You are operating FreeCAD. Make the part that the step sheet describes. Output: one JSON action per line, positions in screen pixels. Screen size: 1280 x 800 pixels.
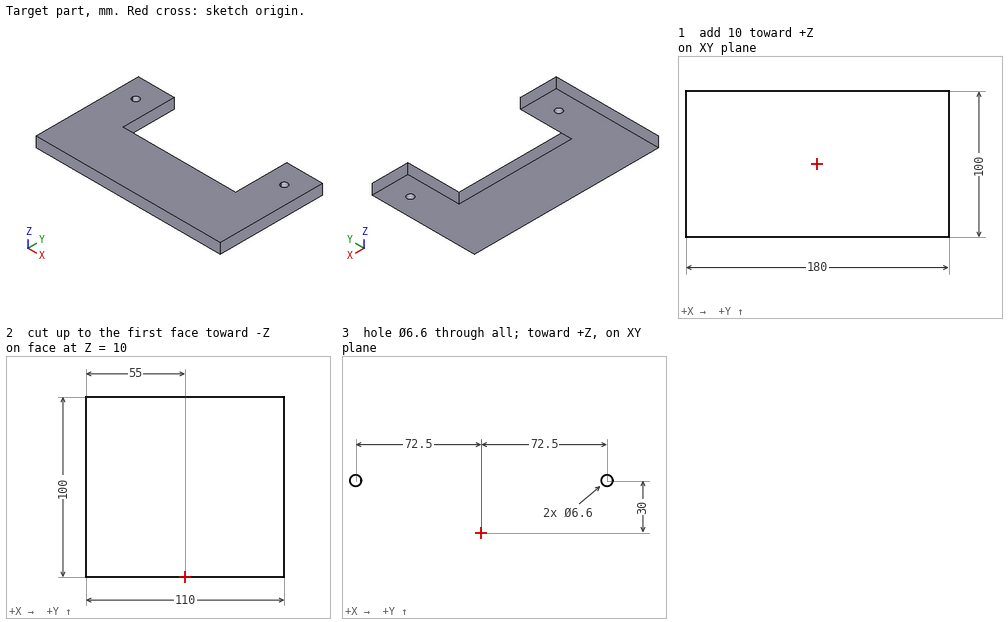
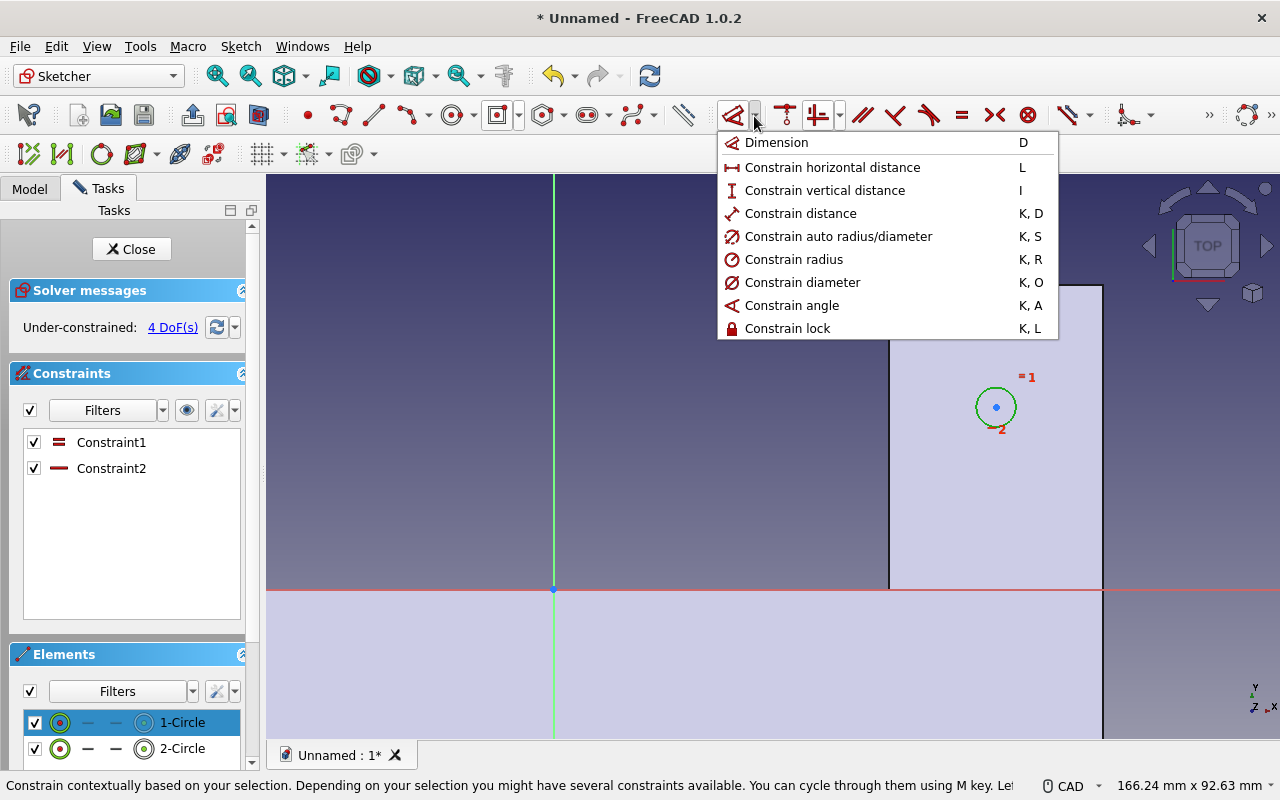
{"action": "left_click", "coordinate": [888, 282]}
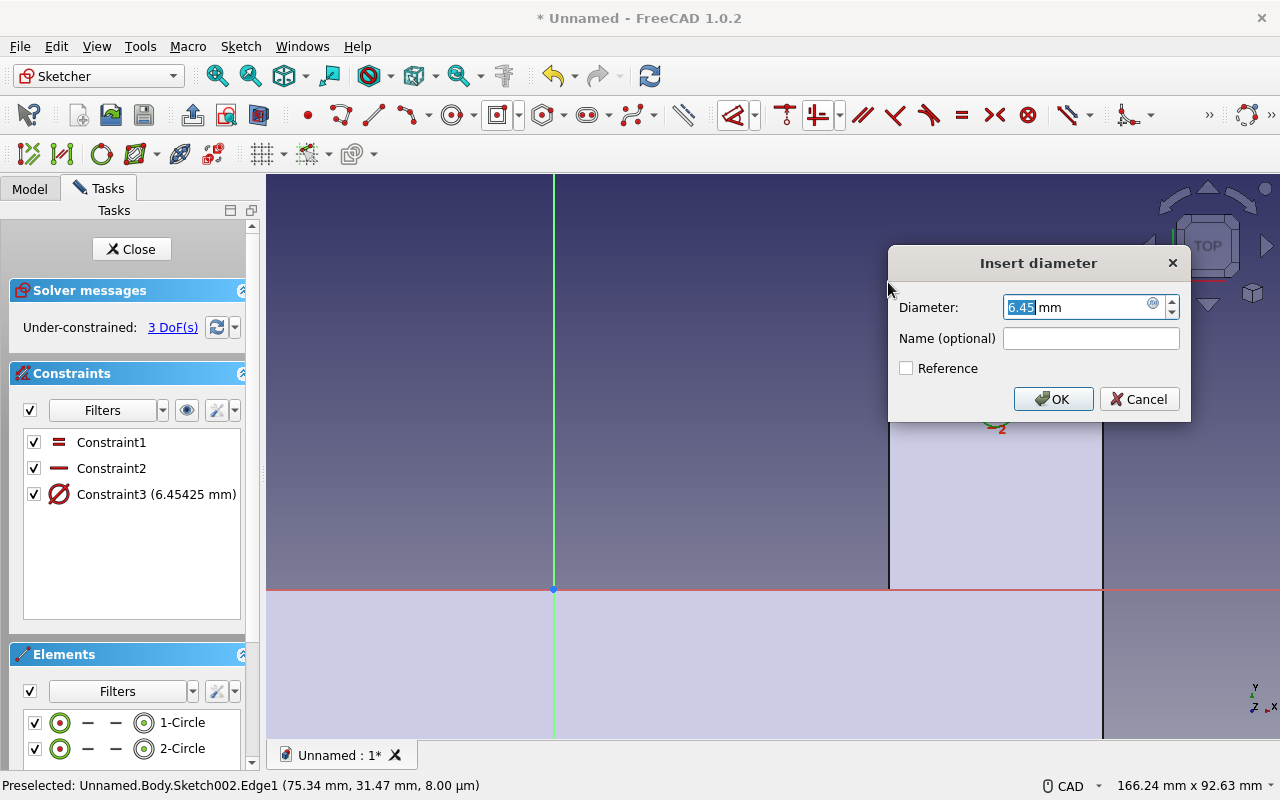
{"action": "type", "text": "6.6"}
{"action": "key", "text": "Return"}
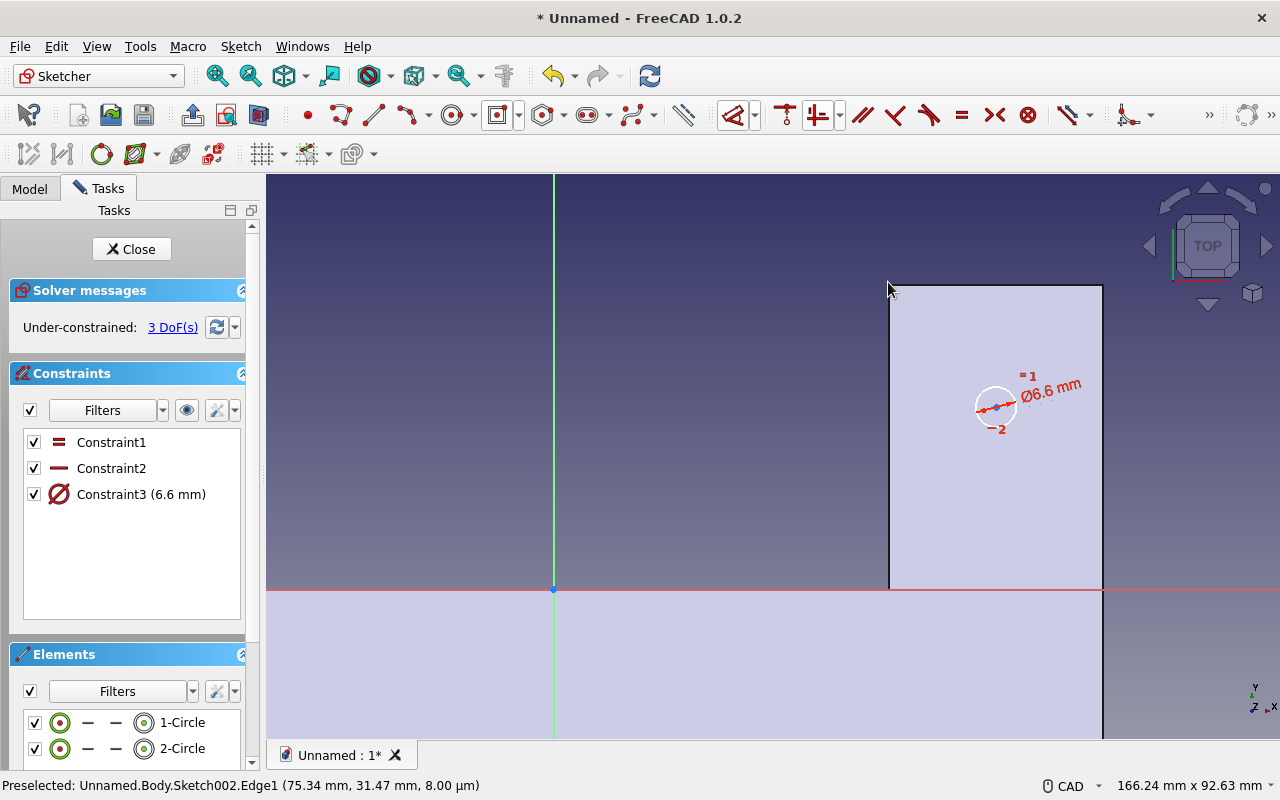
{"action": "left_click", "coordinate": [996, 407]}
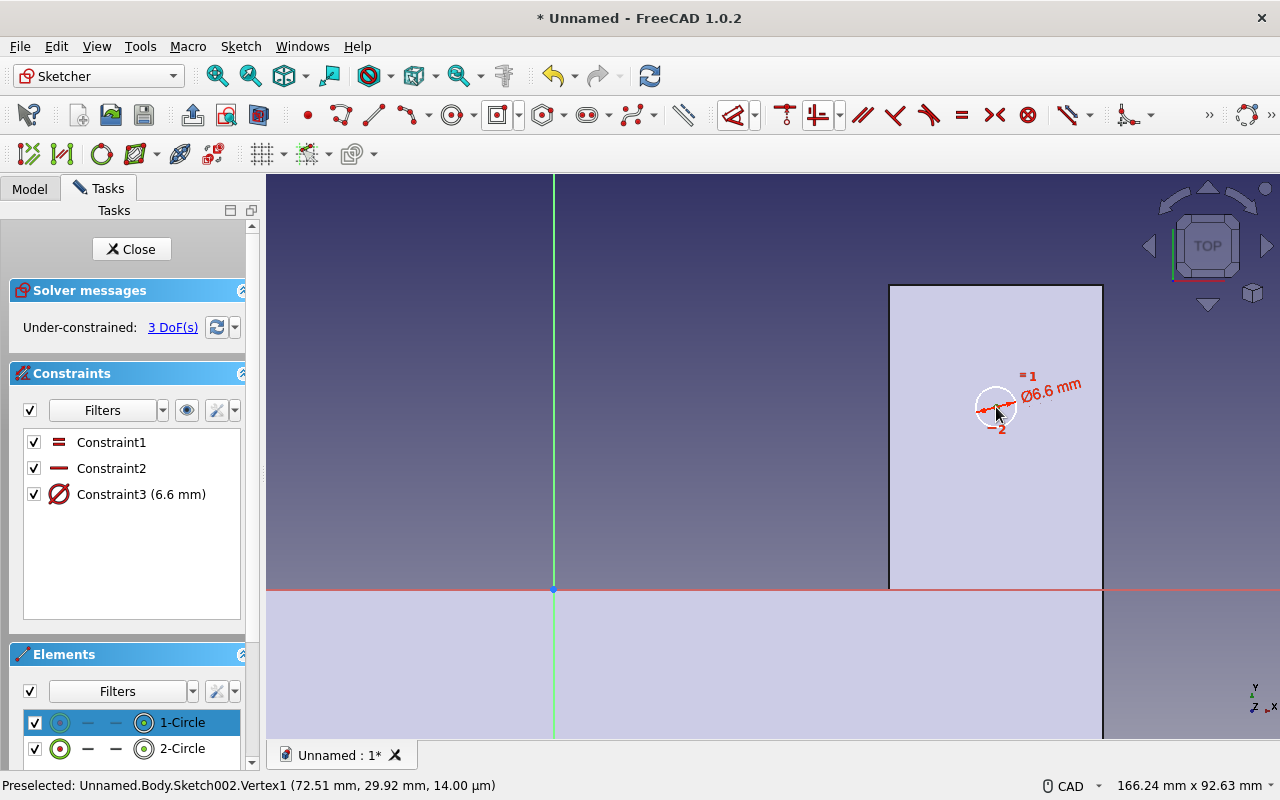
{"action": "key", "text": "i"}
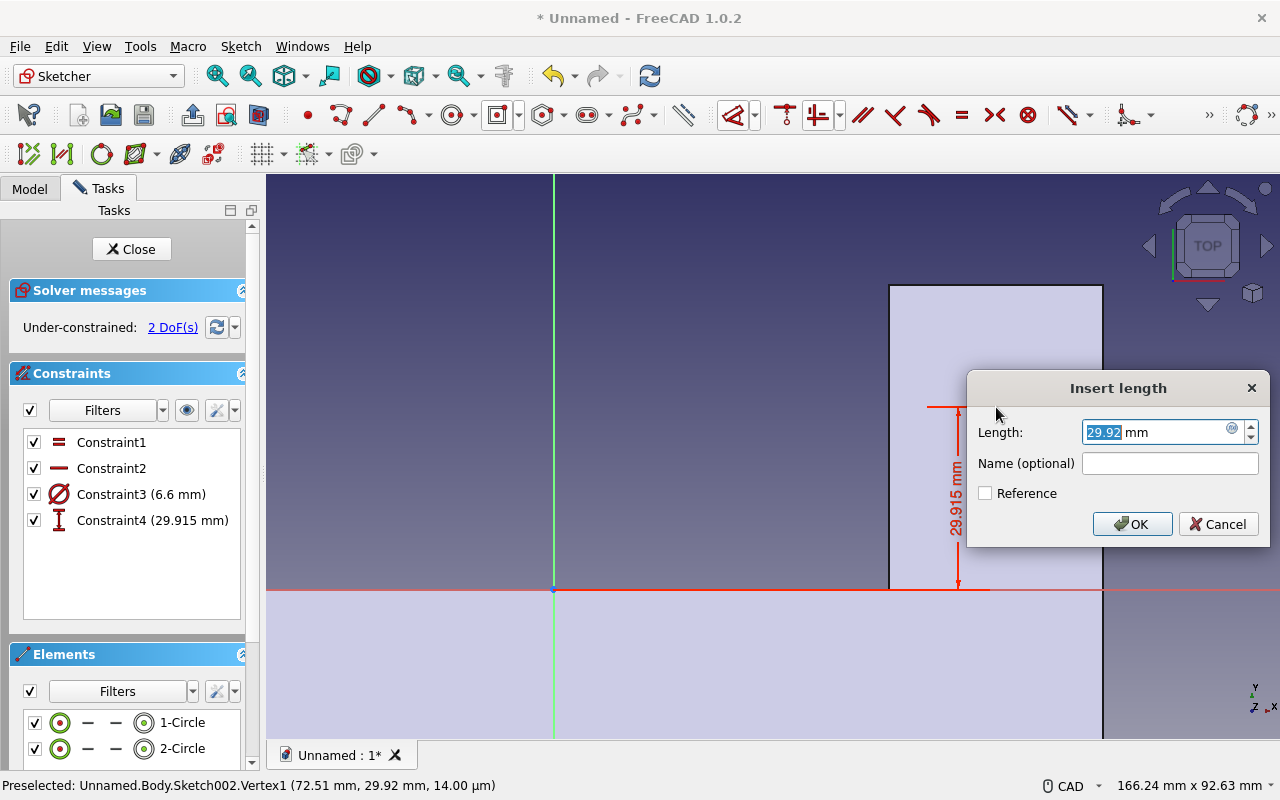
{"action": "type", "text": "30"}
{"action": "key", "text": "Return"}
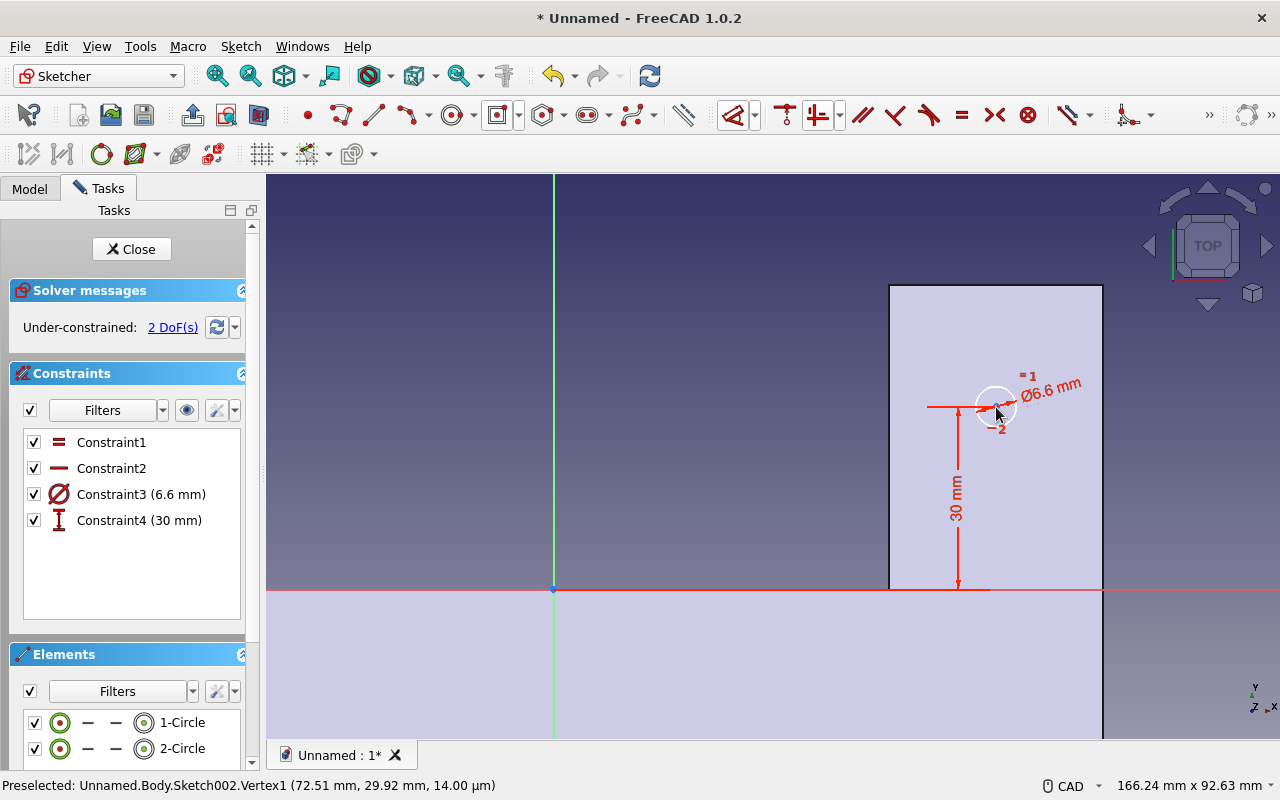
{"action": "left_click", "coordinate": [996, 407]}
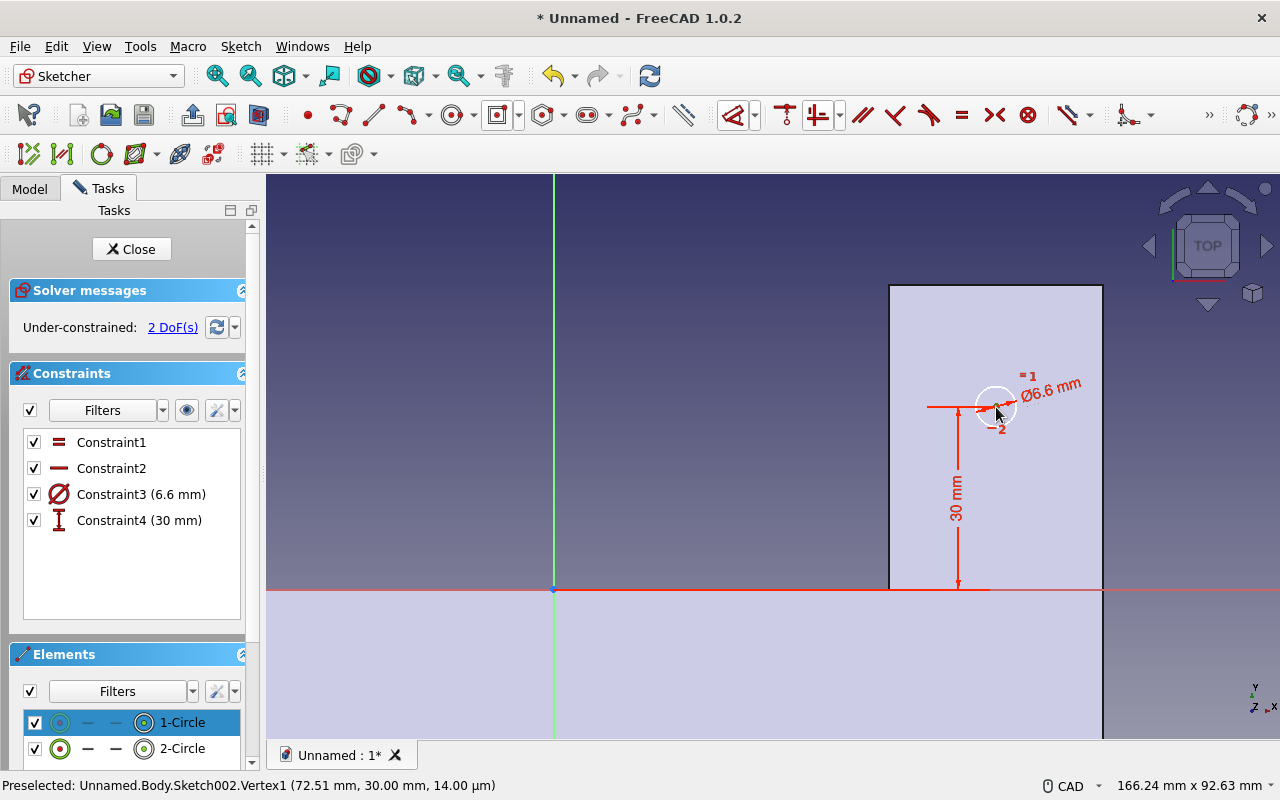
{"action": "left_click", "coordinate": [754, 116]}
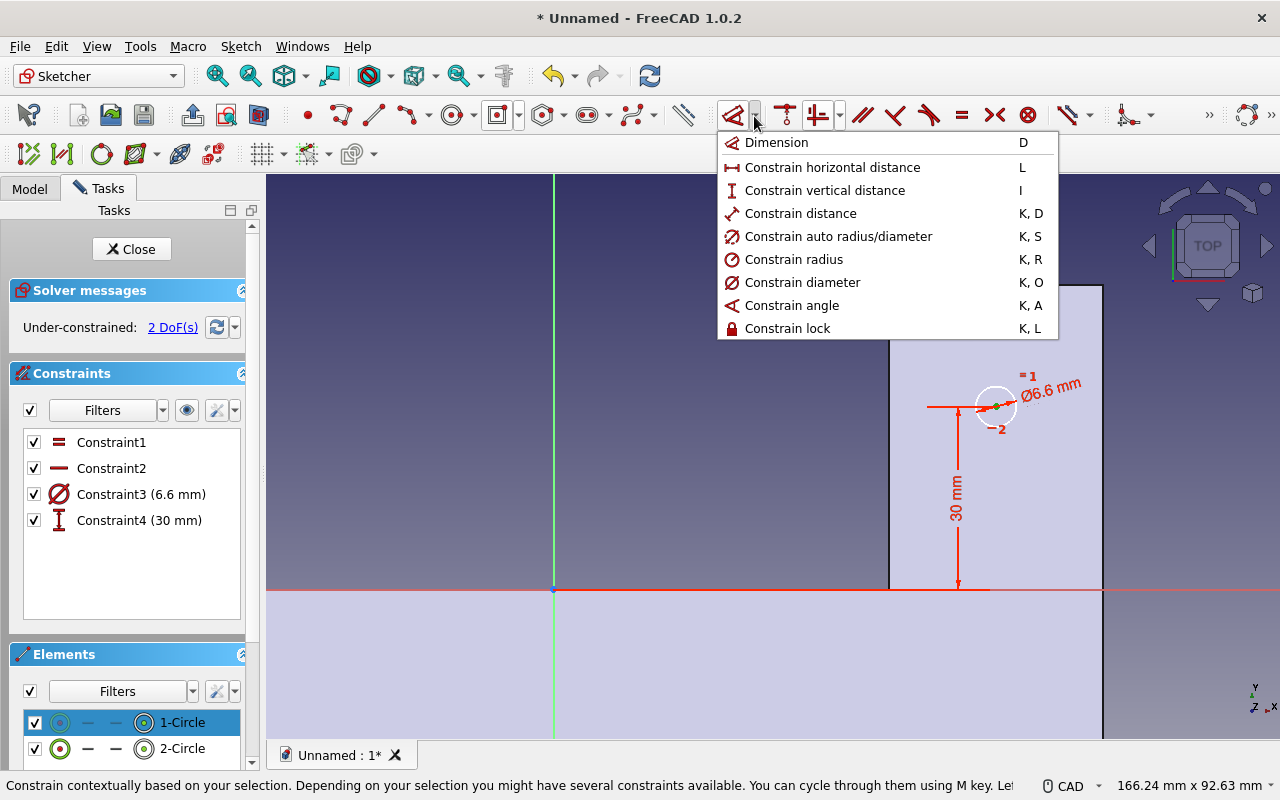
{"action": "left_click", "coordinate": [888, 168]}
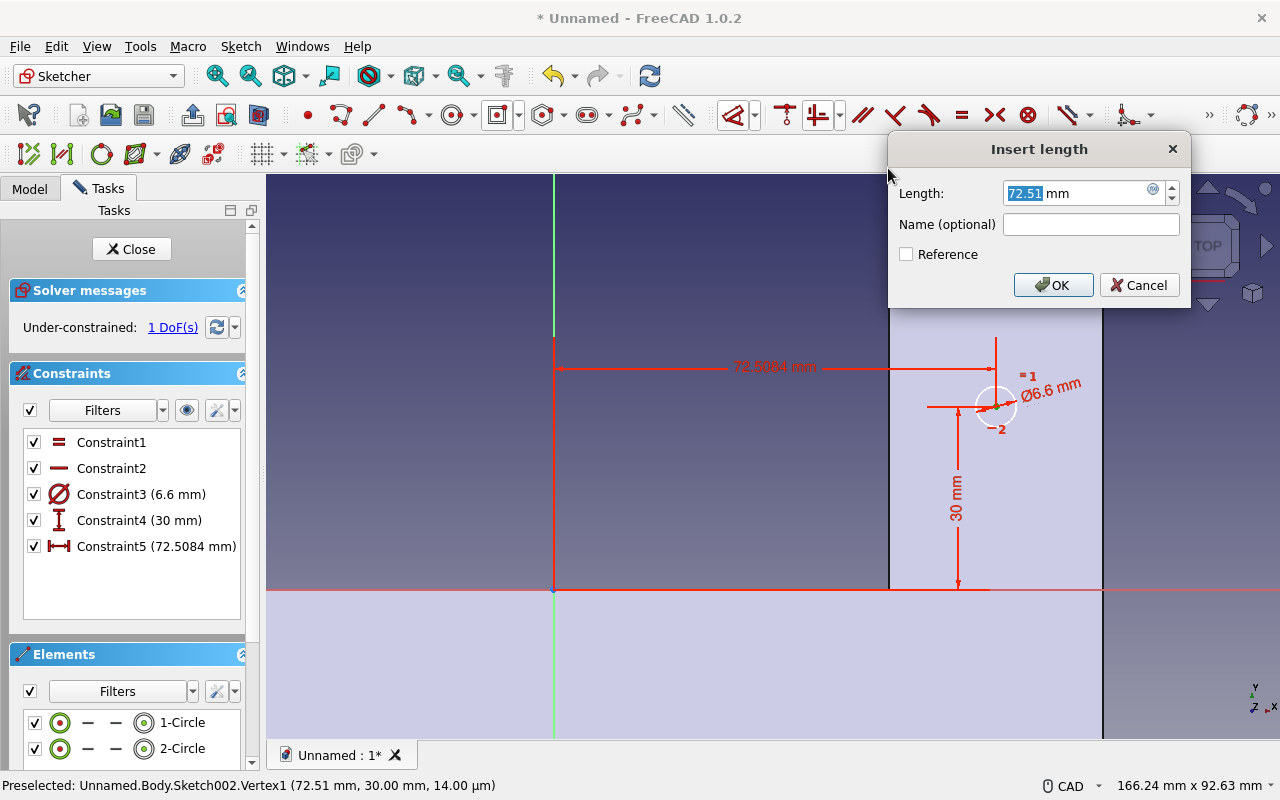
{"action": "type", "text": "72.5"}
{"action": "key", "text": "Return"}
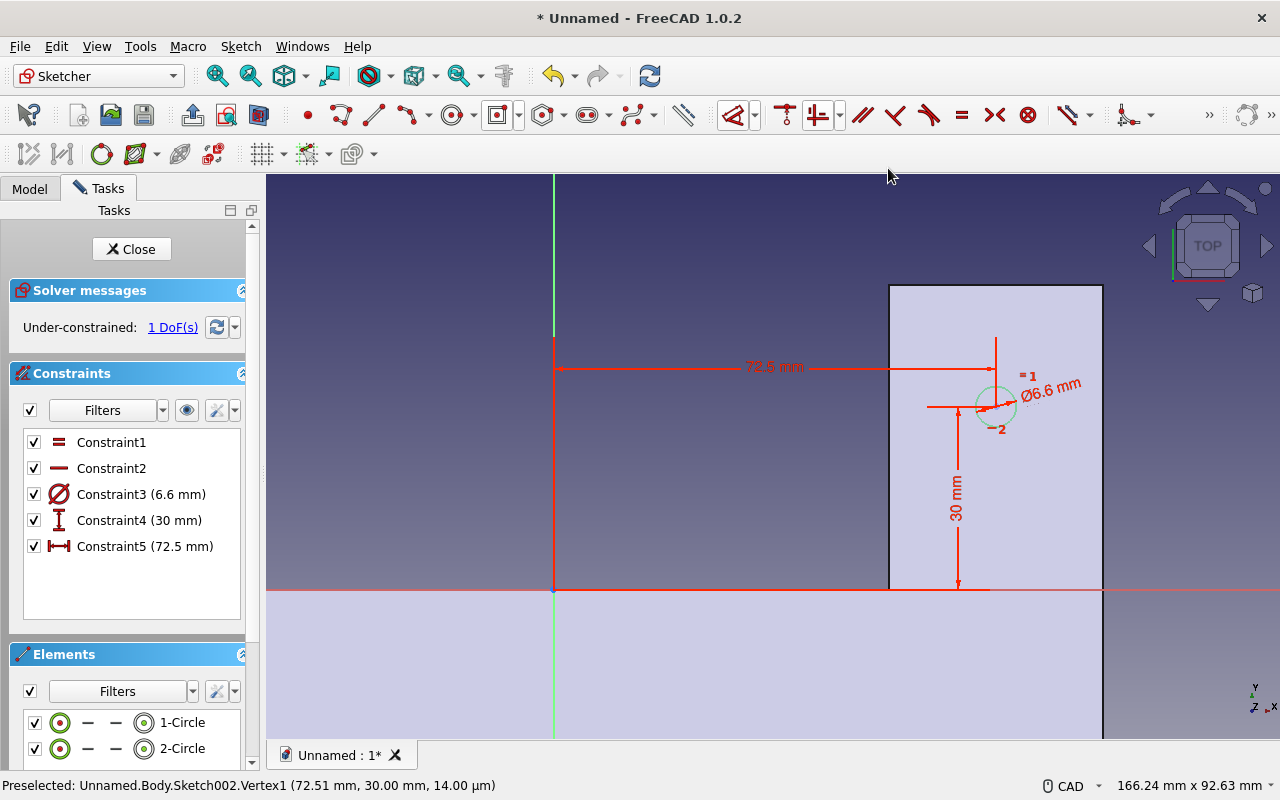
{"action": "scroll", "coordinate": [1011, 392], "scroll_direction": "down", "scroll_amount": 2}